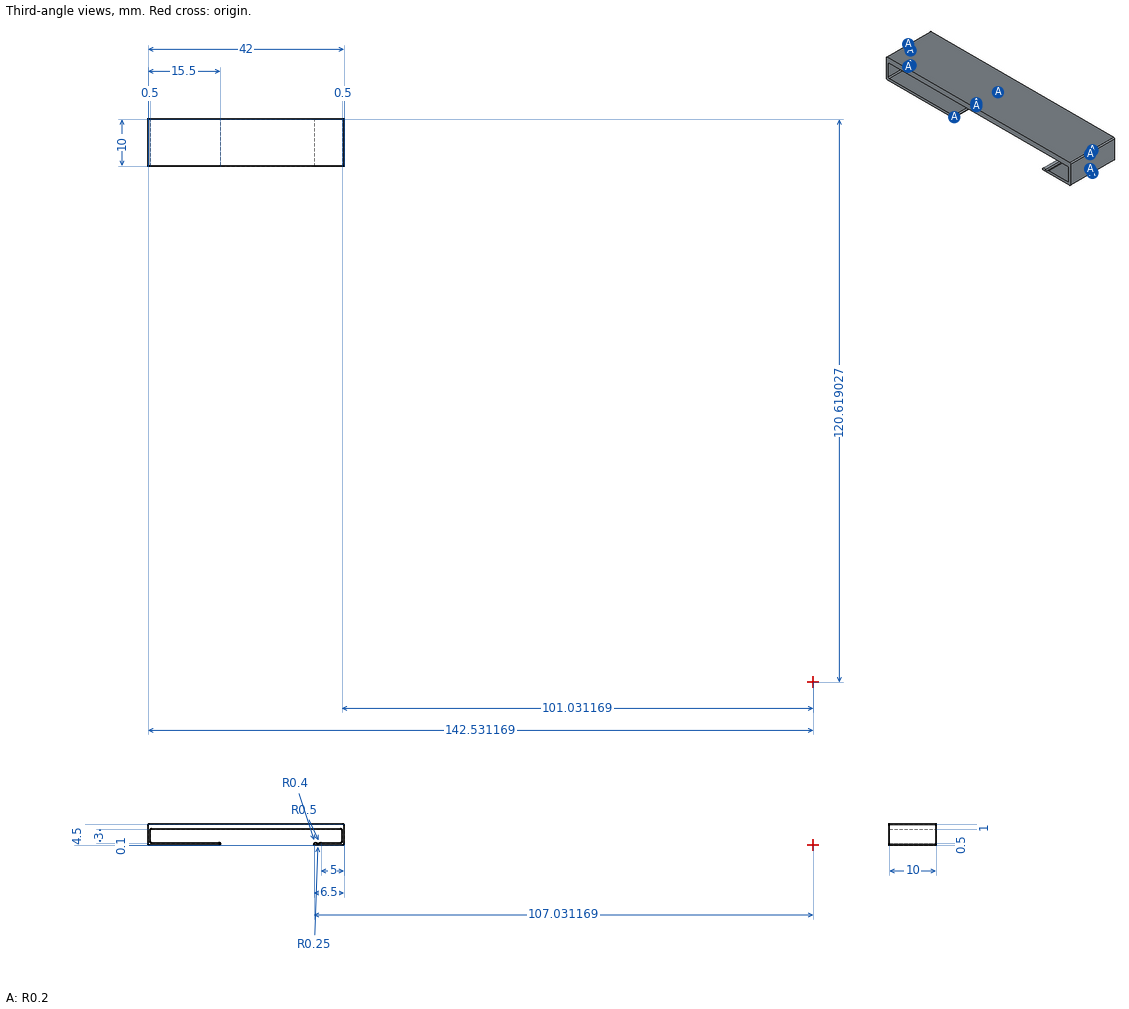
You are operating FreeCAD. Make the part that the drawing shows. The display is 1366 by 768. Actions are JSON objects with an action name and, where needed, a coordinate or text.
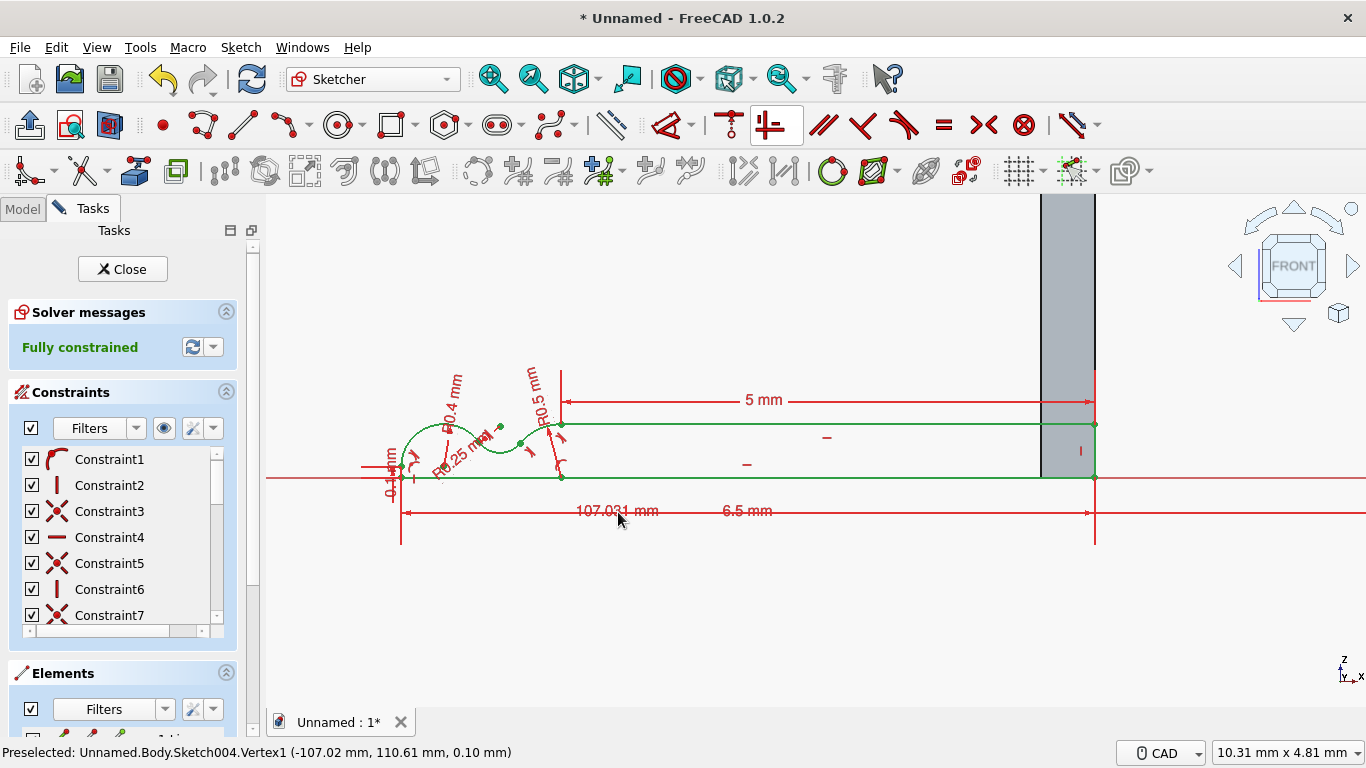
{"action": "left_click", "coordinate": [123, 269]}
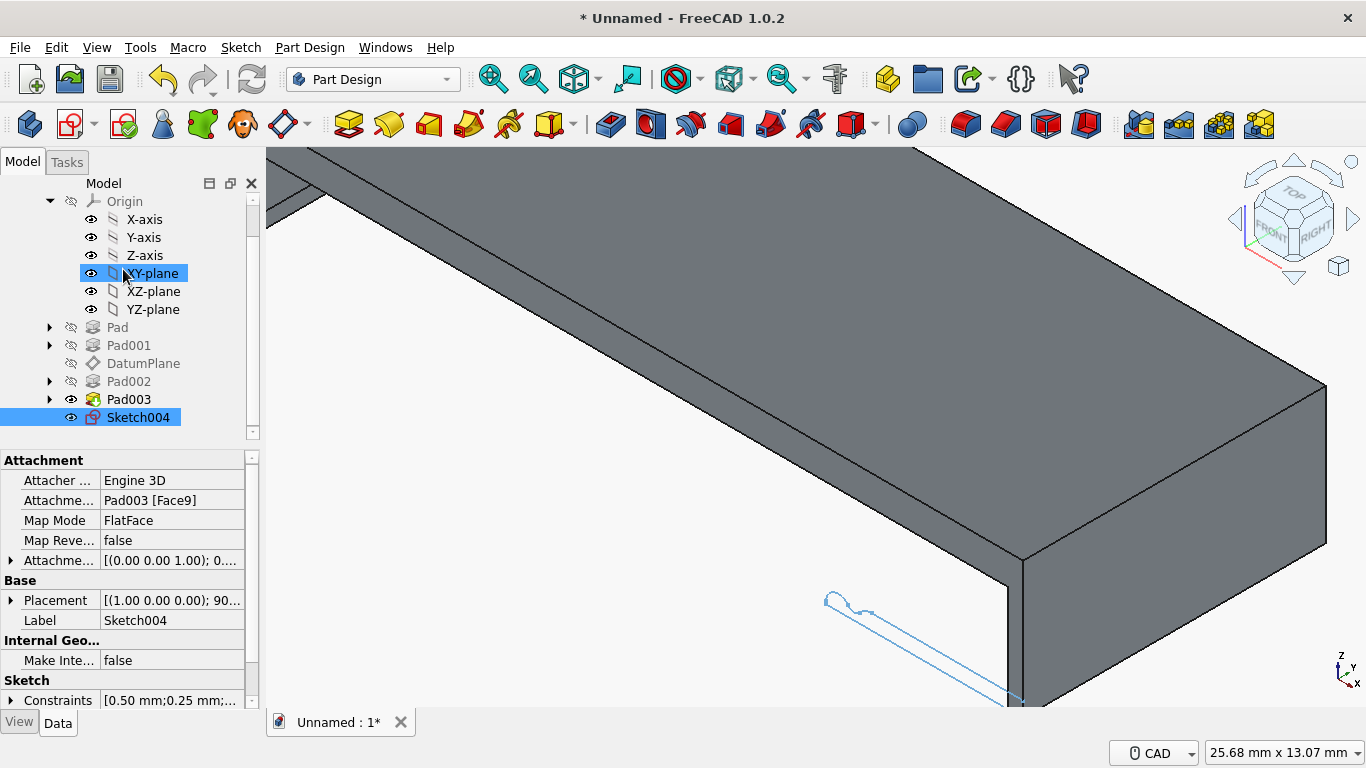
{"action": "left_click", "coordinate": [350, 124]}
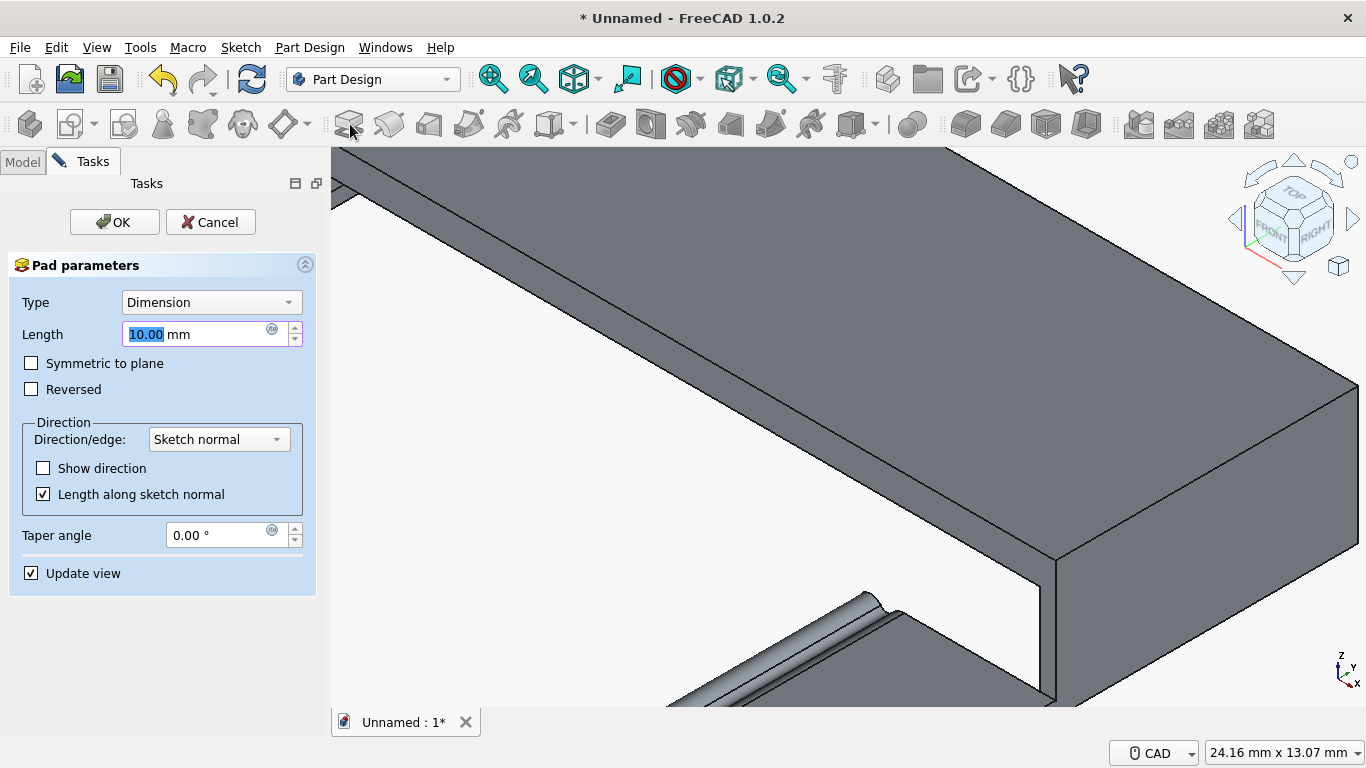
{"action": "type", "text": "10"}
{"action": "key", "text": "Tab"}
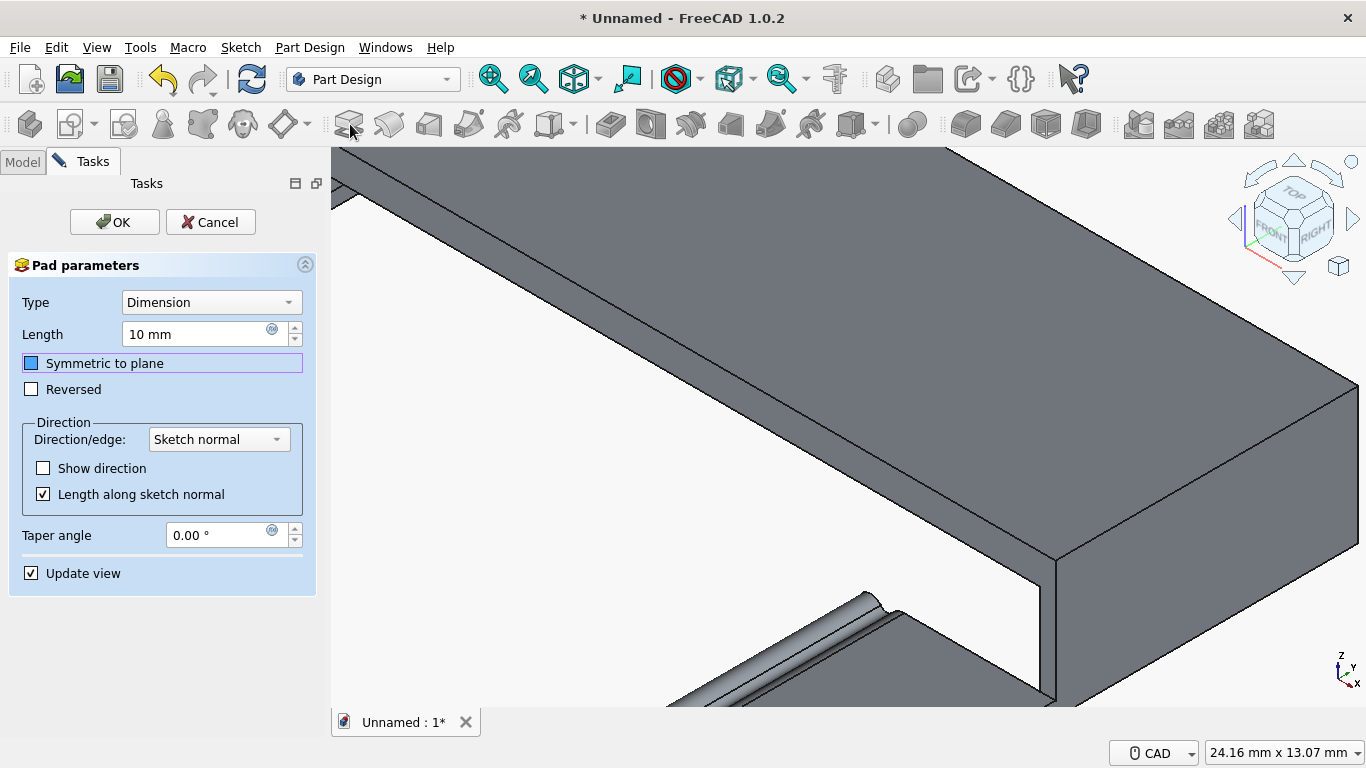
{"action": "left_click", "coordinate": [30, 389]}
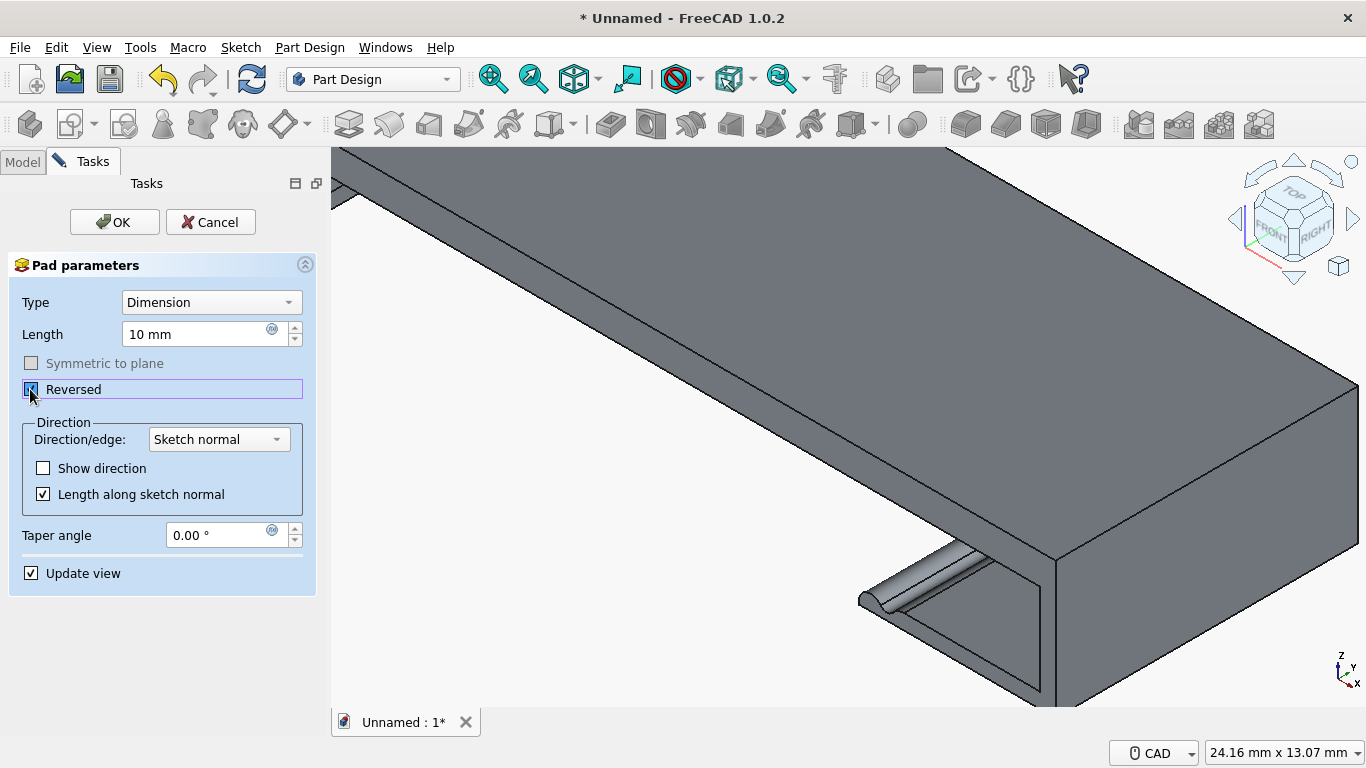
{"action": "left_click", "coordinate": [115, 222]}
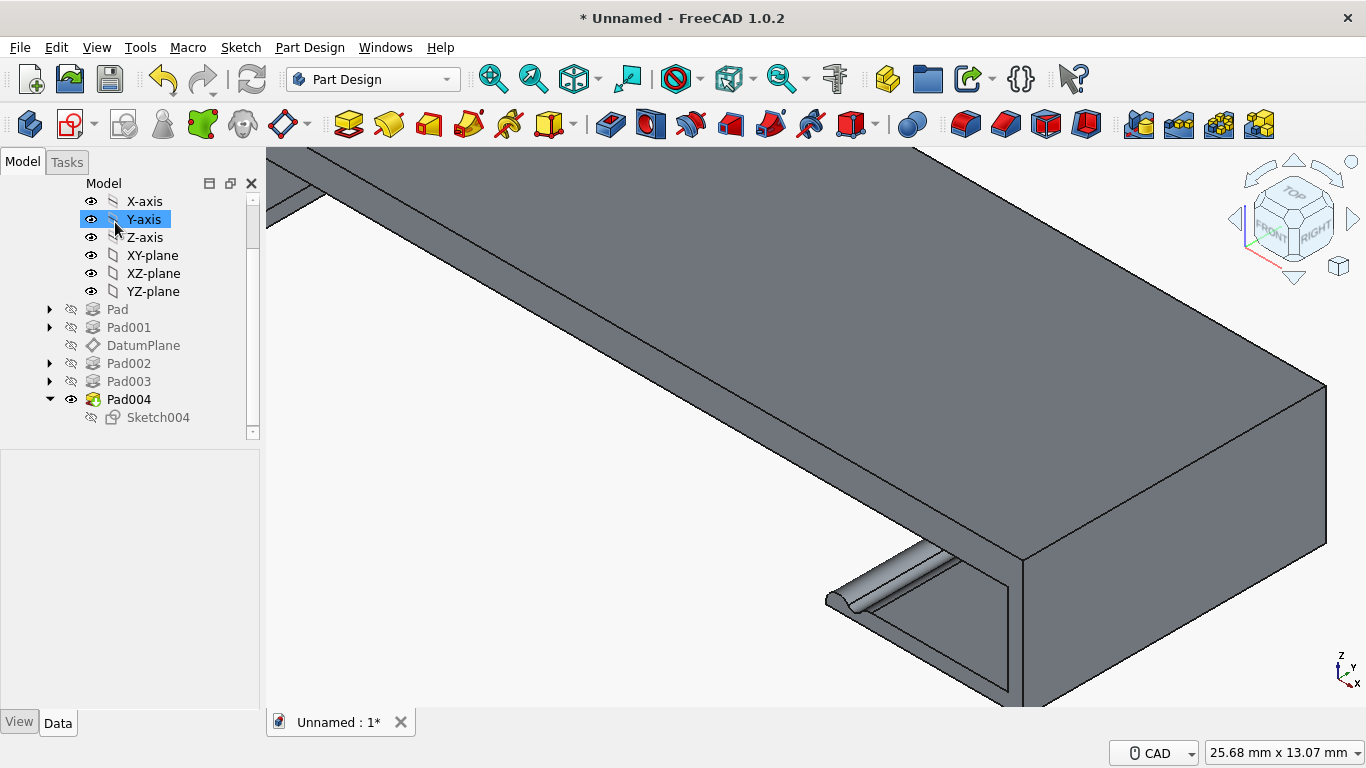
{"action": "left_click", "coordinate": [494, 80]}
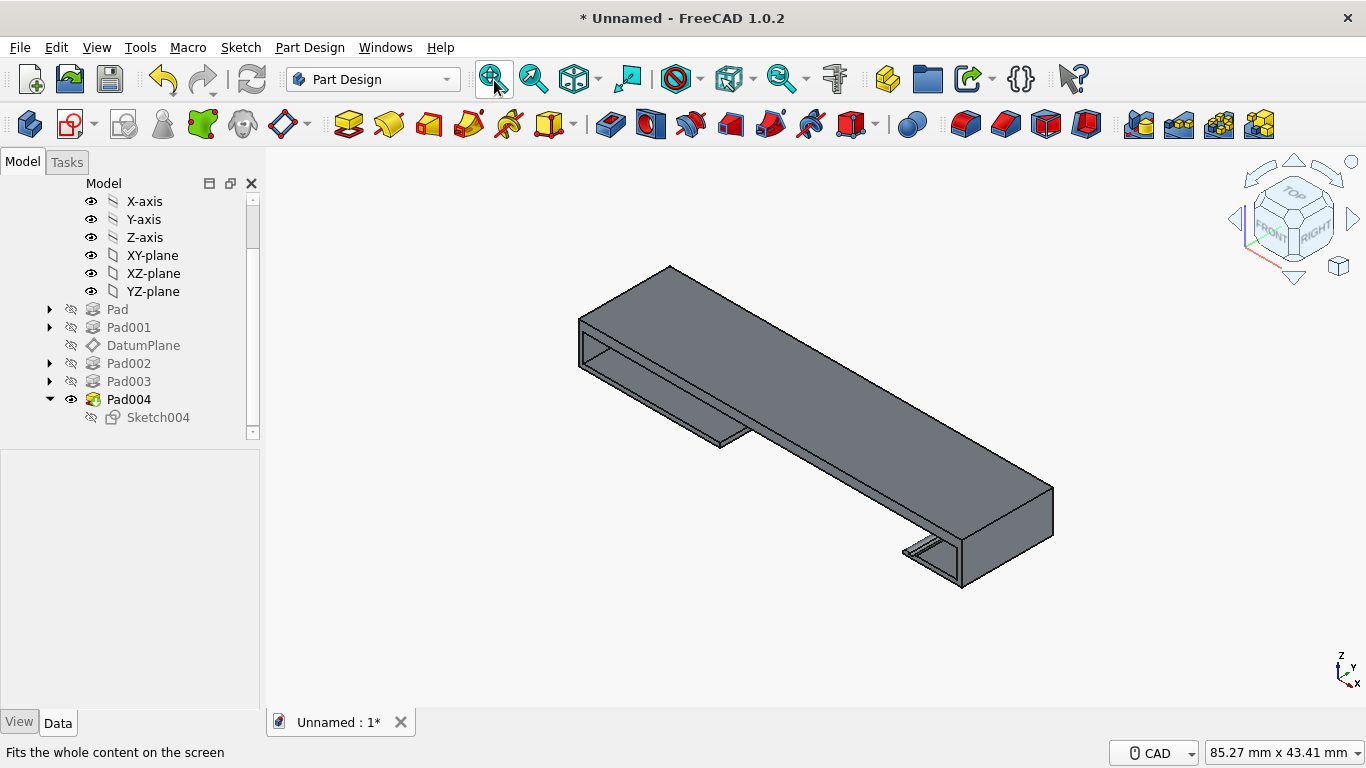
{"action": "left_click", "coordinate": [1008, 513]}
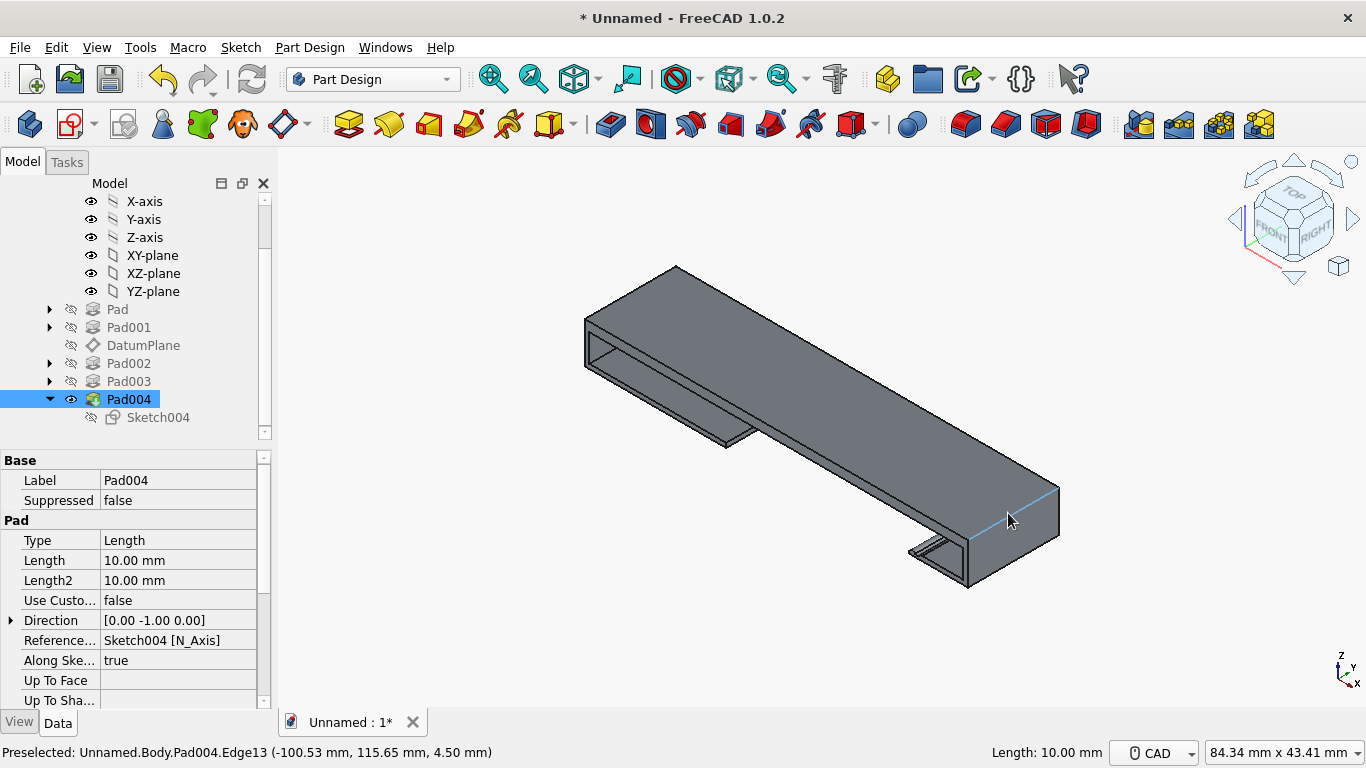
{"action": "scroll", "coordinate": [811, 396], "scroll_direction": "up", "scroll_amount": 7}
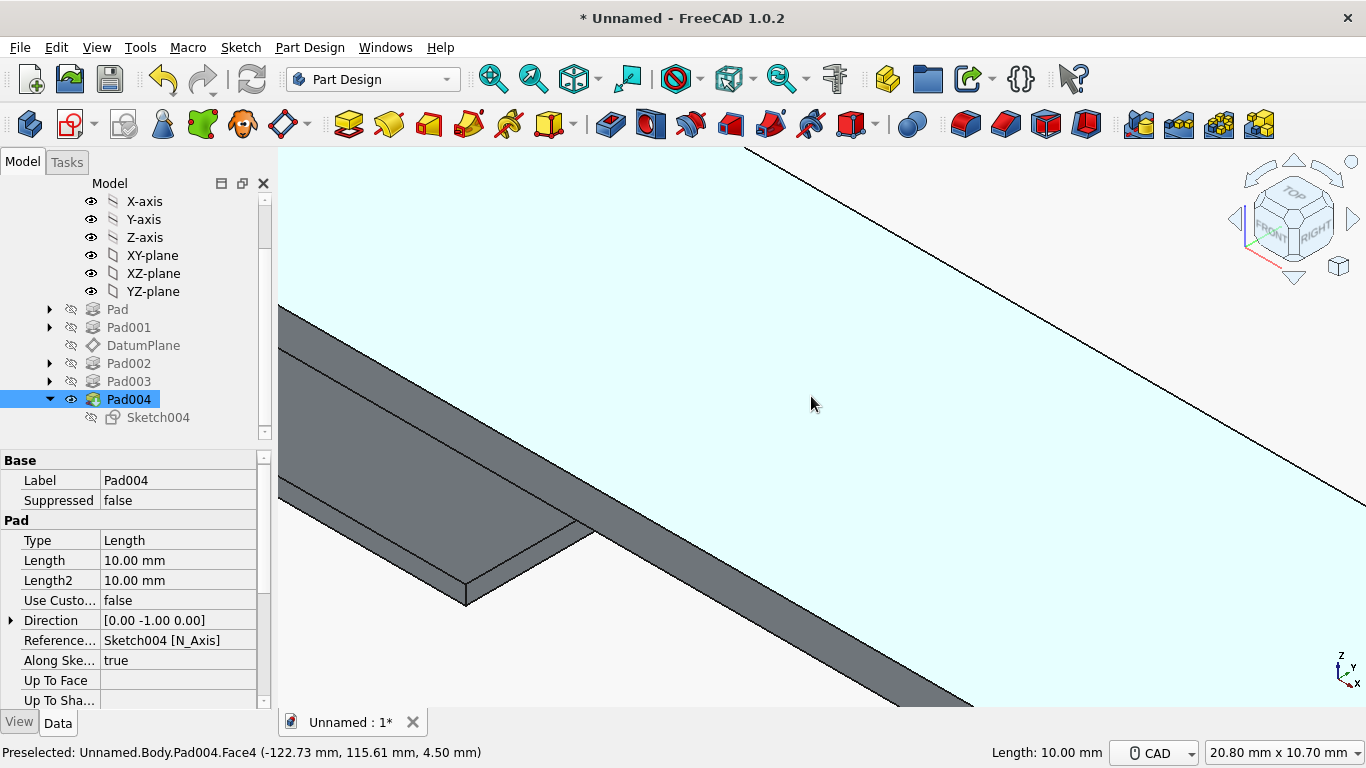
{"action": "left_click", "coordinate": [492, 579], "text": "ctrl"}